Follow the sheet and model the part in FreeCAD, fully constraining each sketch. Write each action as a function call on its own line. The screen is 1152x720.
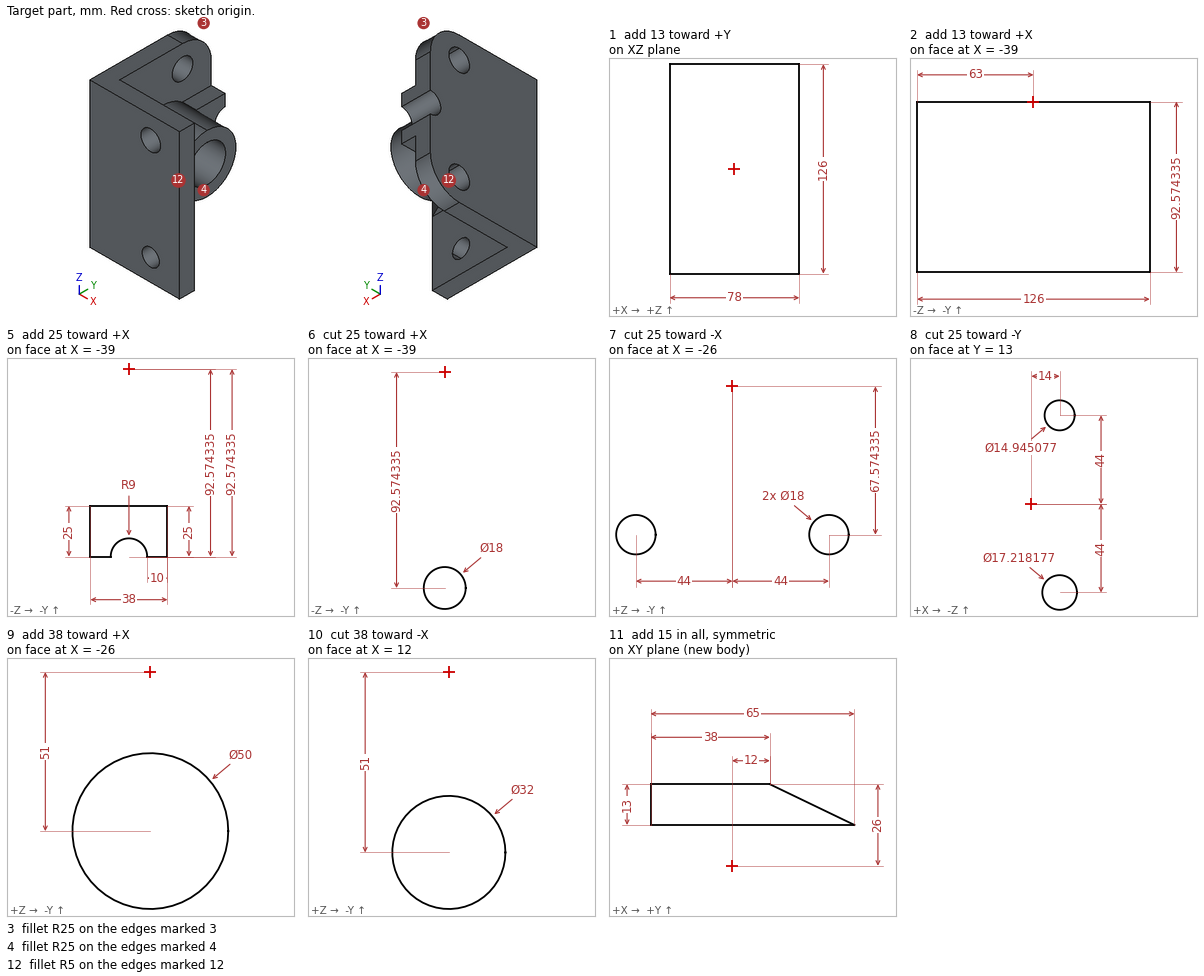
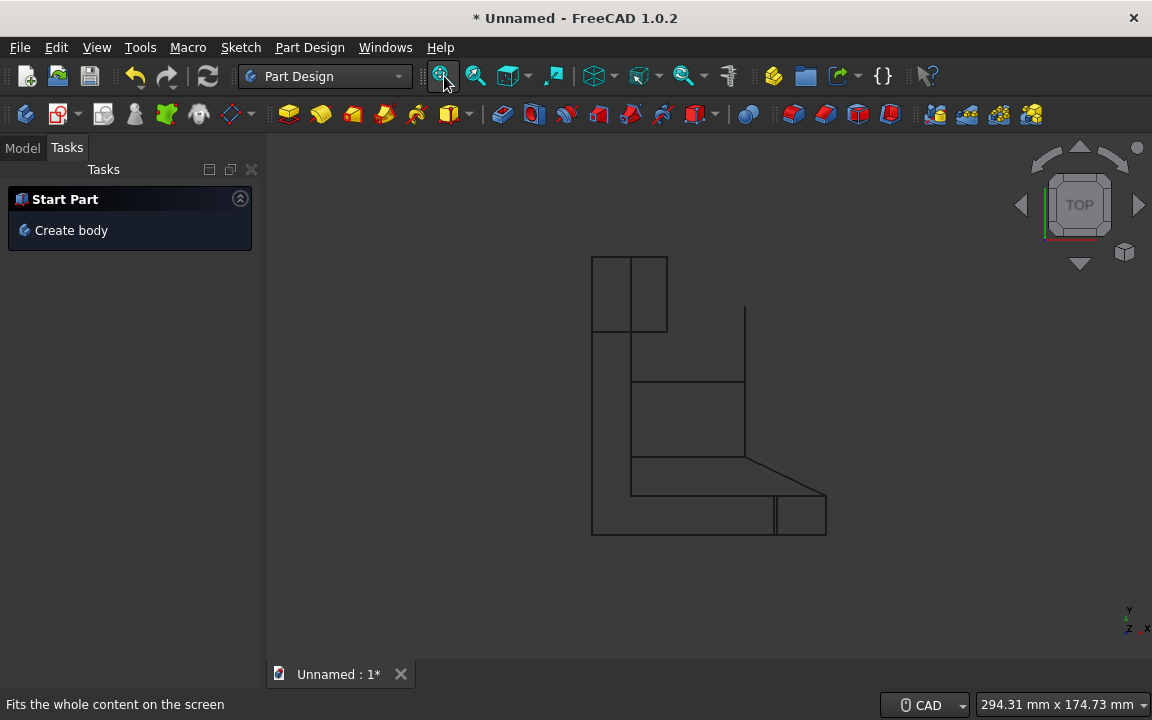
key(v)
key(f)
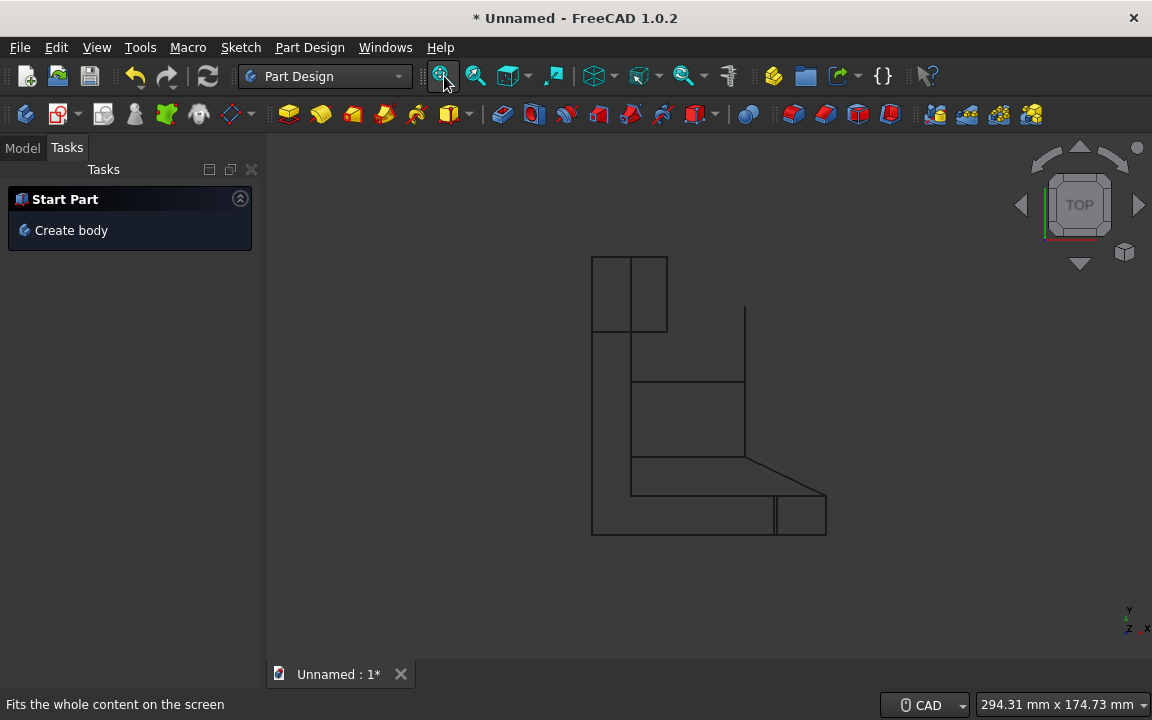
key(1)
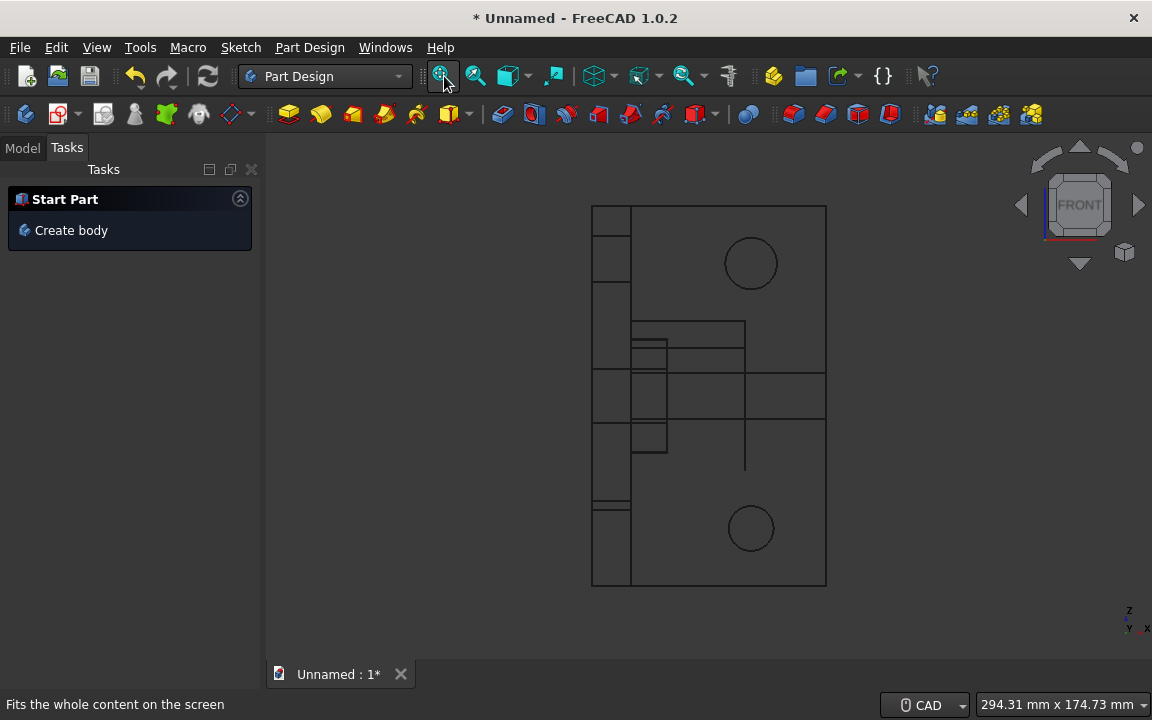
click(444, 76)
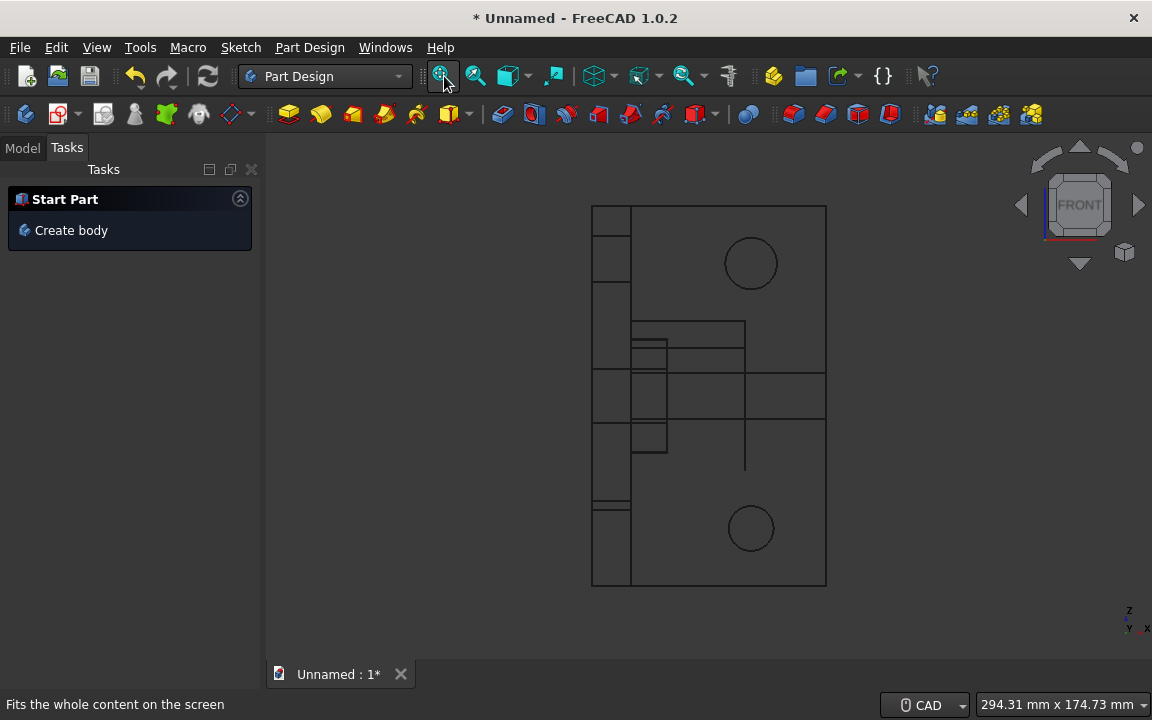
click(745, 395)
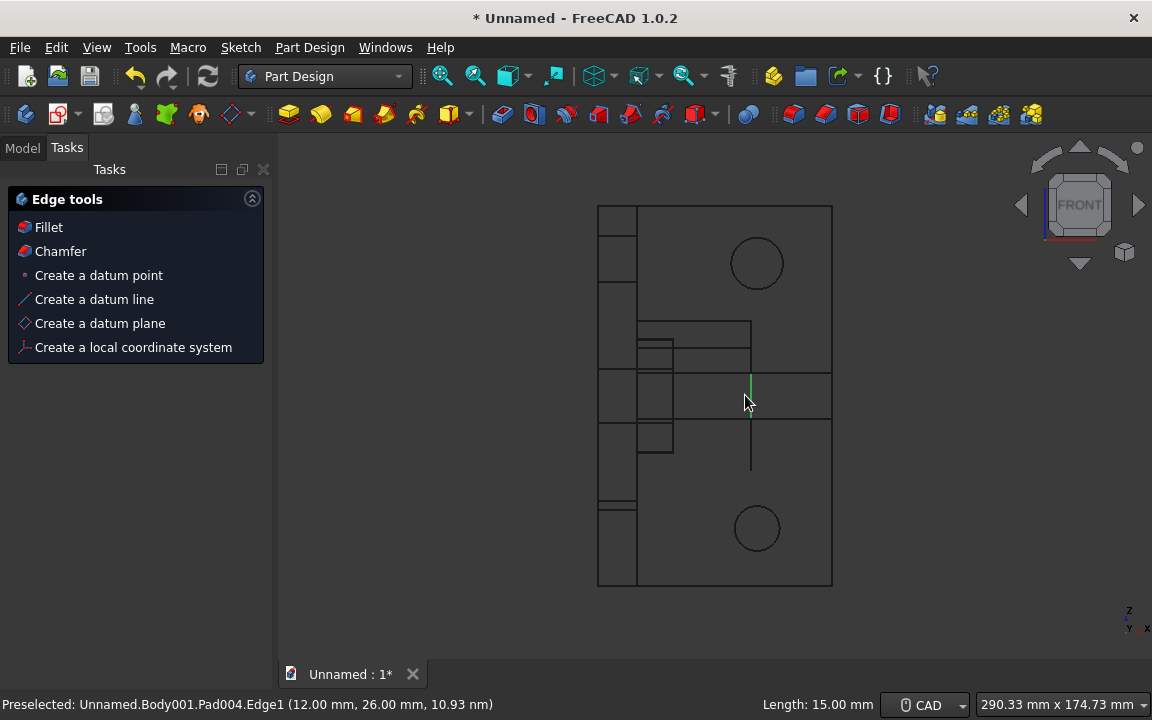
key(v)
key(1)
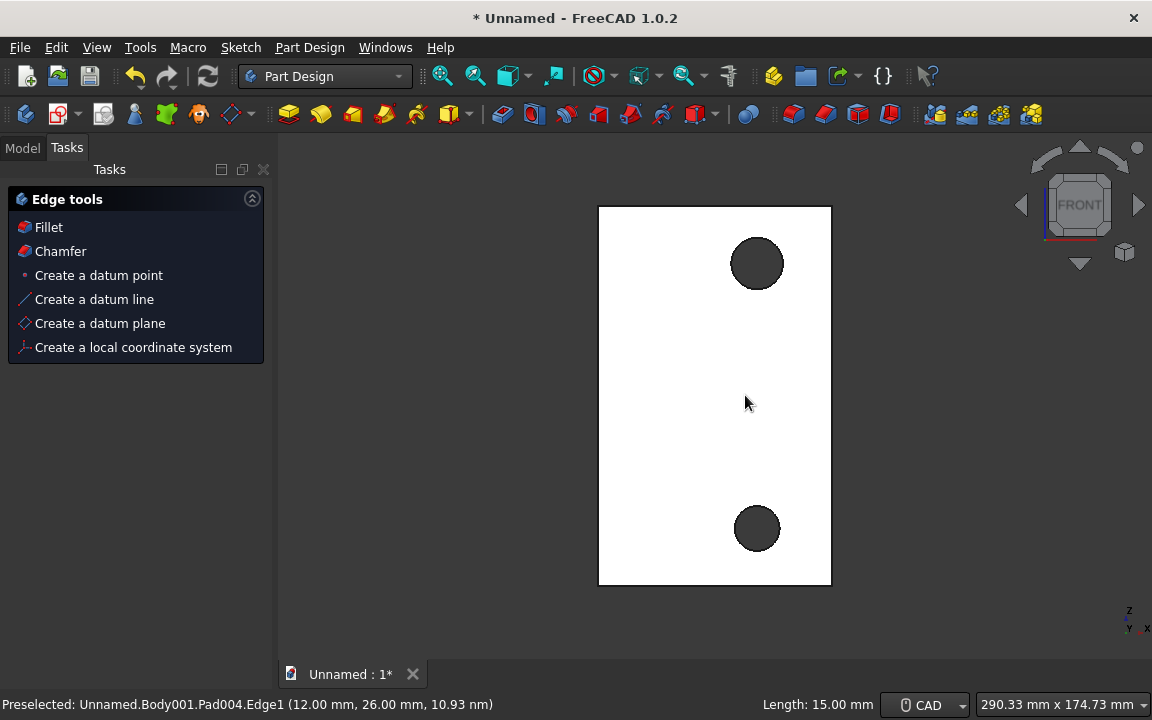
click(794, 114)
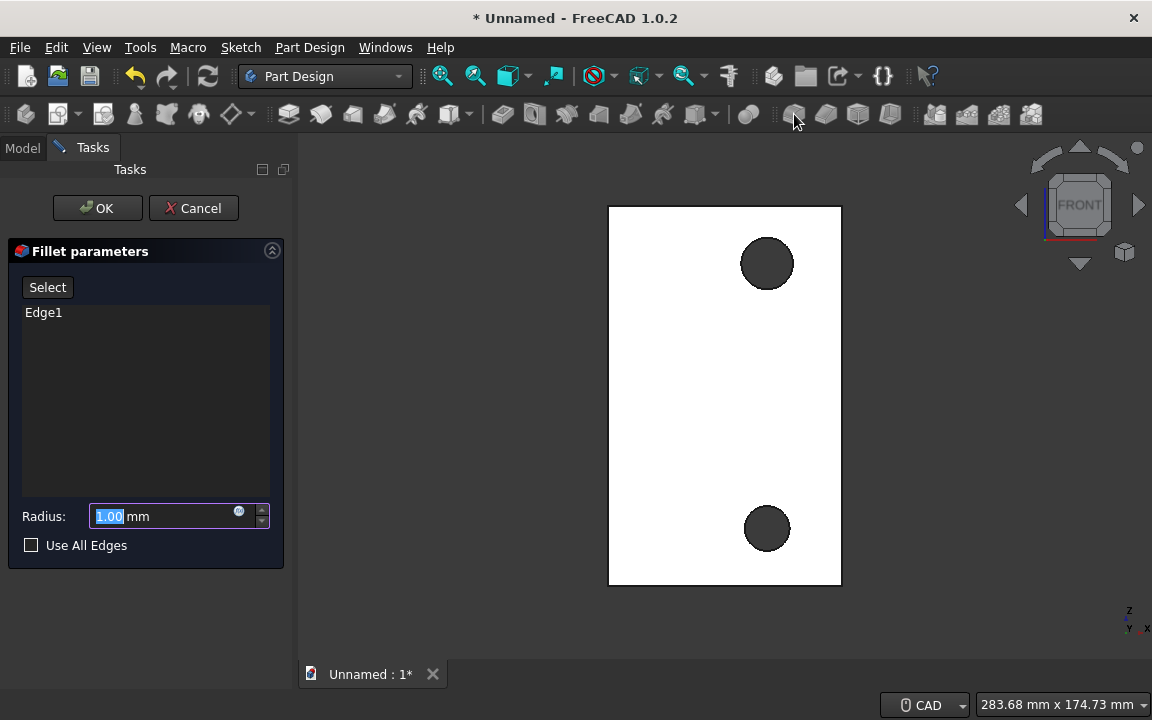
text(5)
key(Tab)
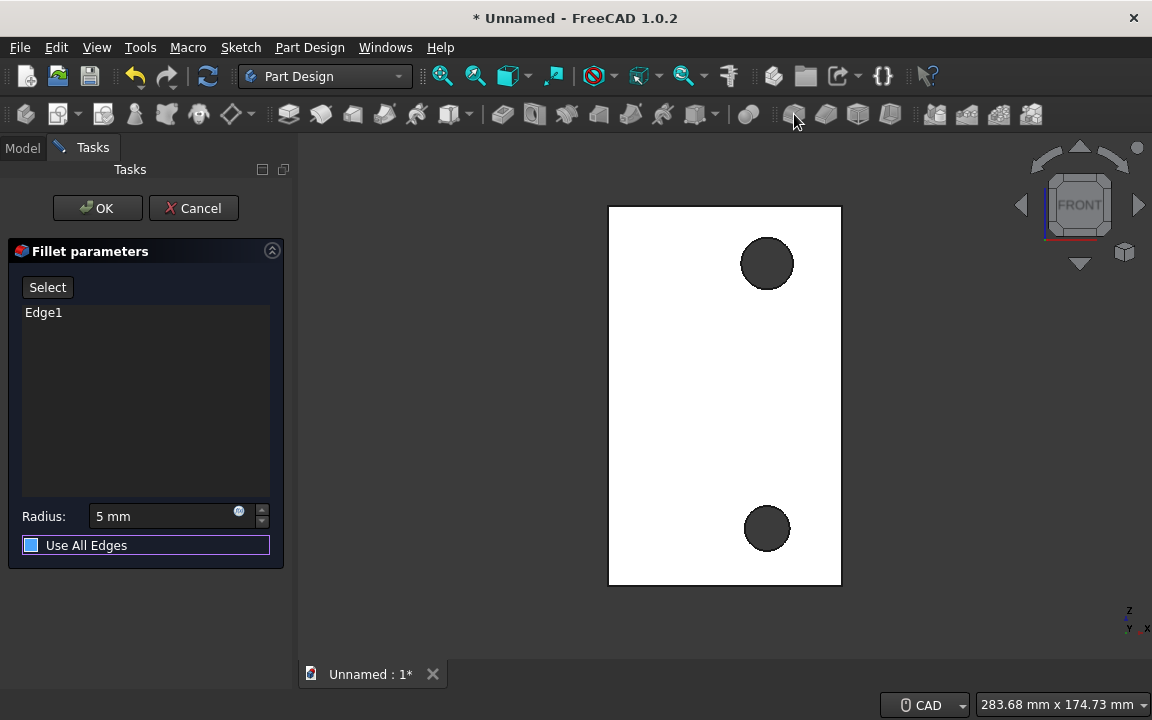
click(98, 208)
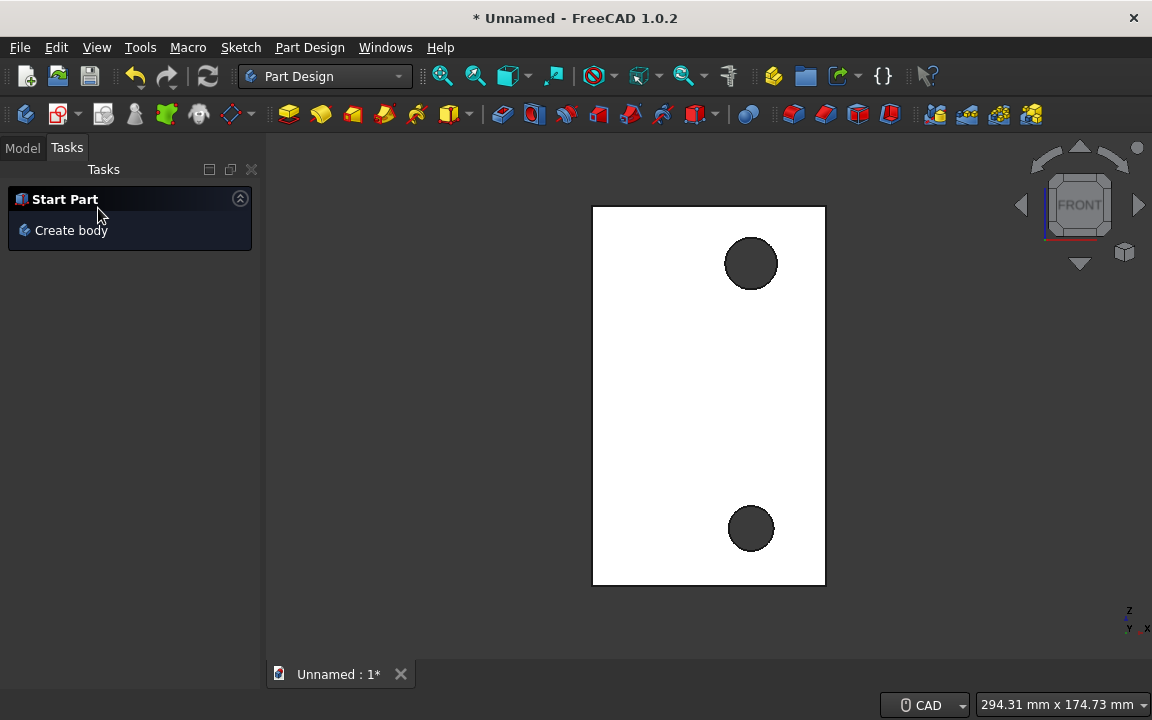
key(0)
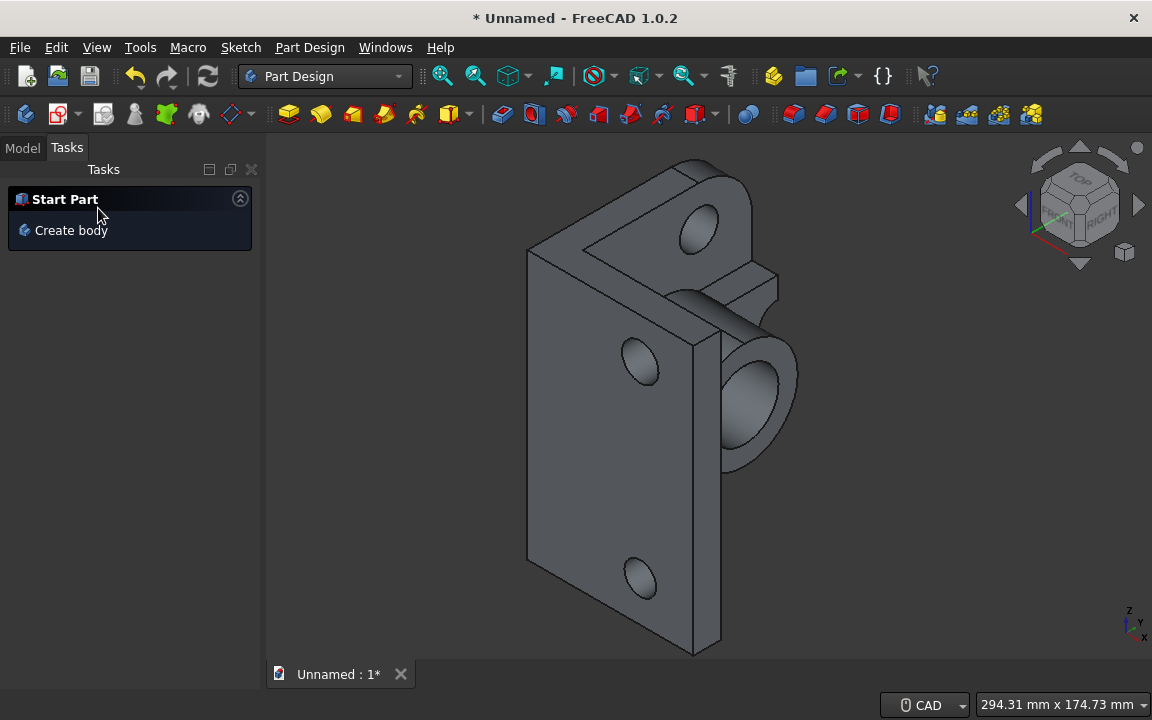
key(v)
key(f)